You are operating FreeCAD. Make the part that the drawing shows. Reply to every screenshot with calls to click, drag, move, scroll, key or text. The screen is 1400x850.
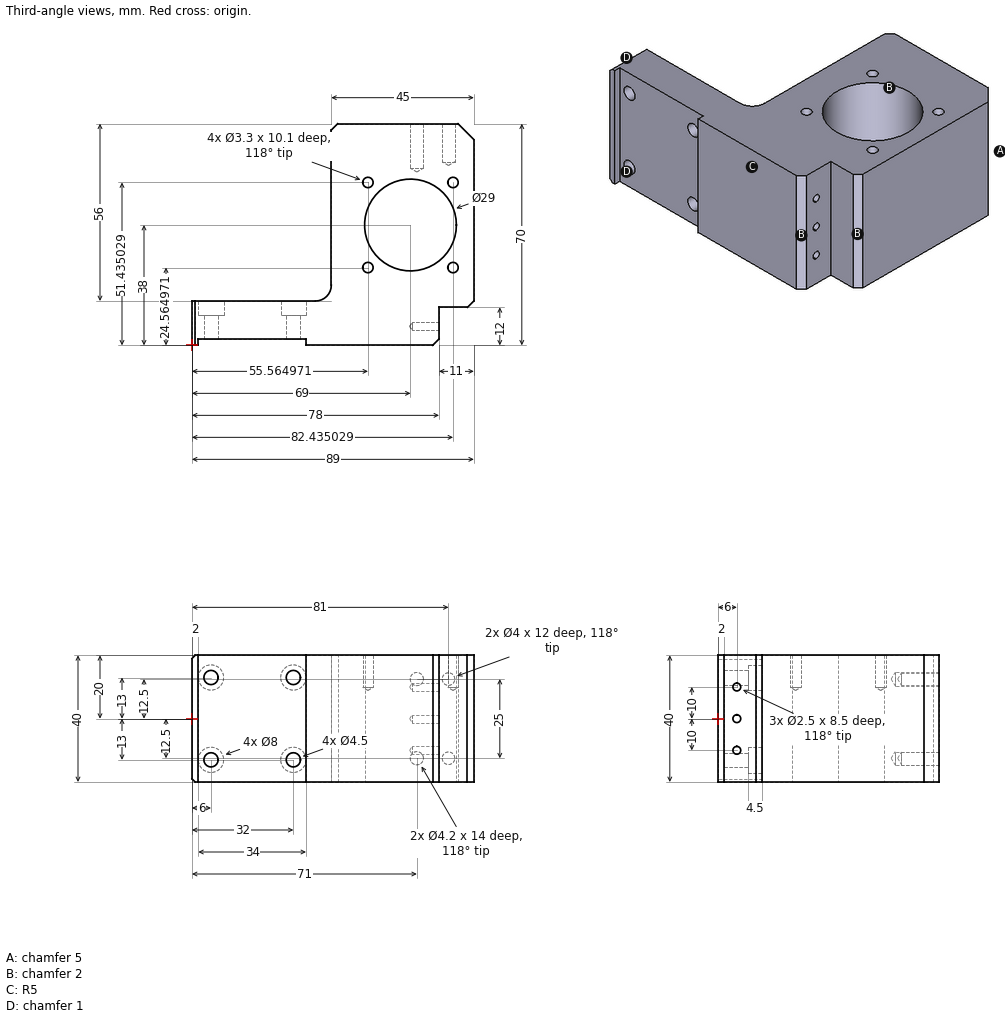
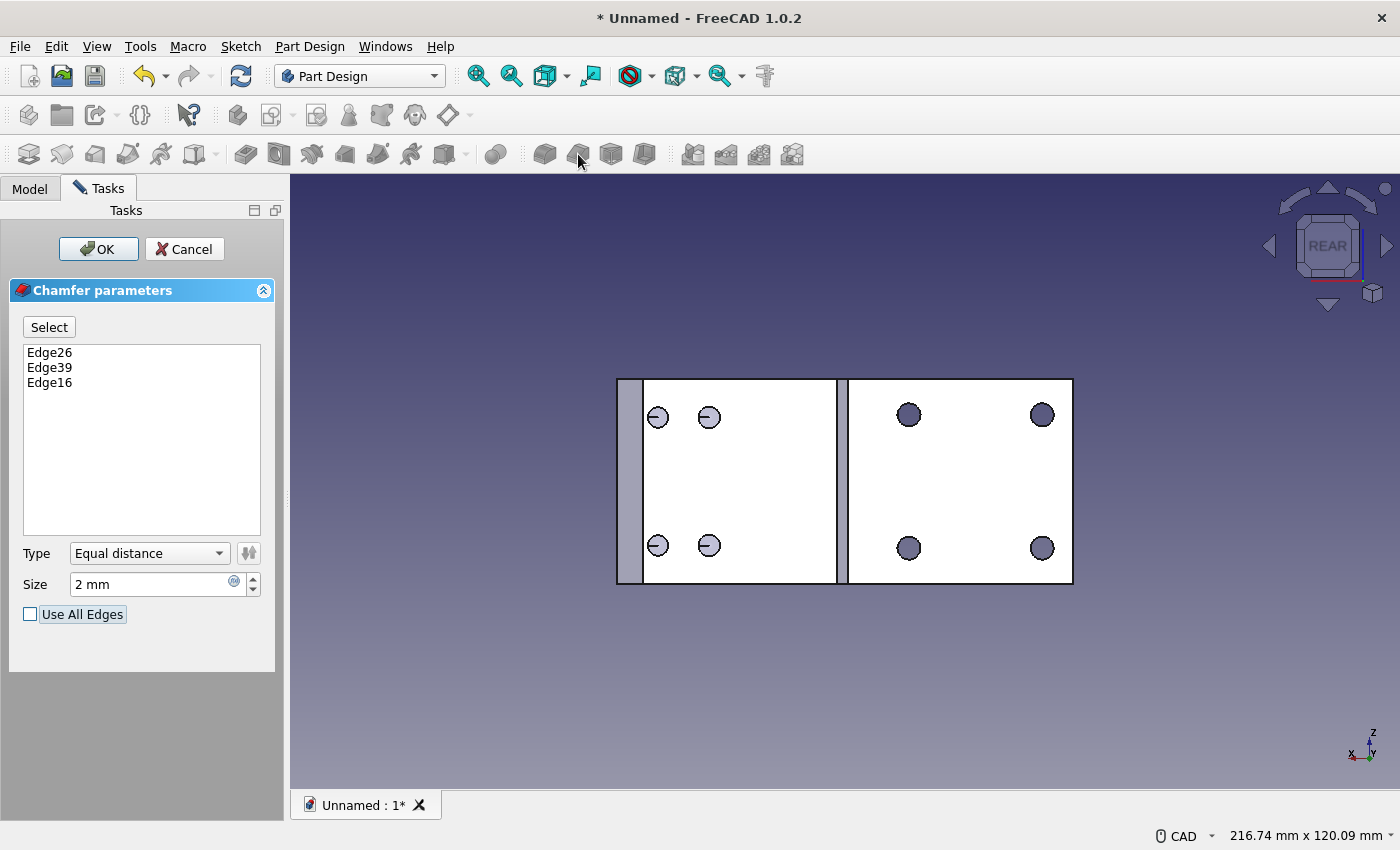
click(99, 249)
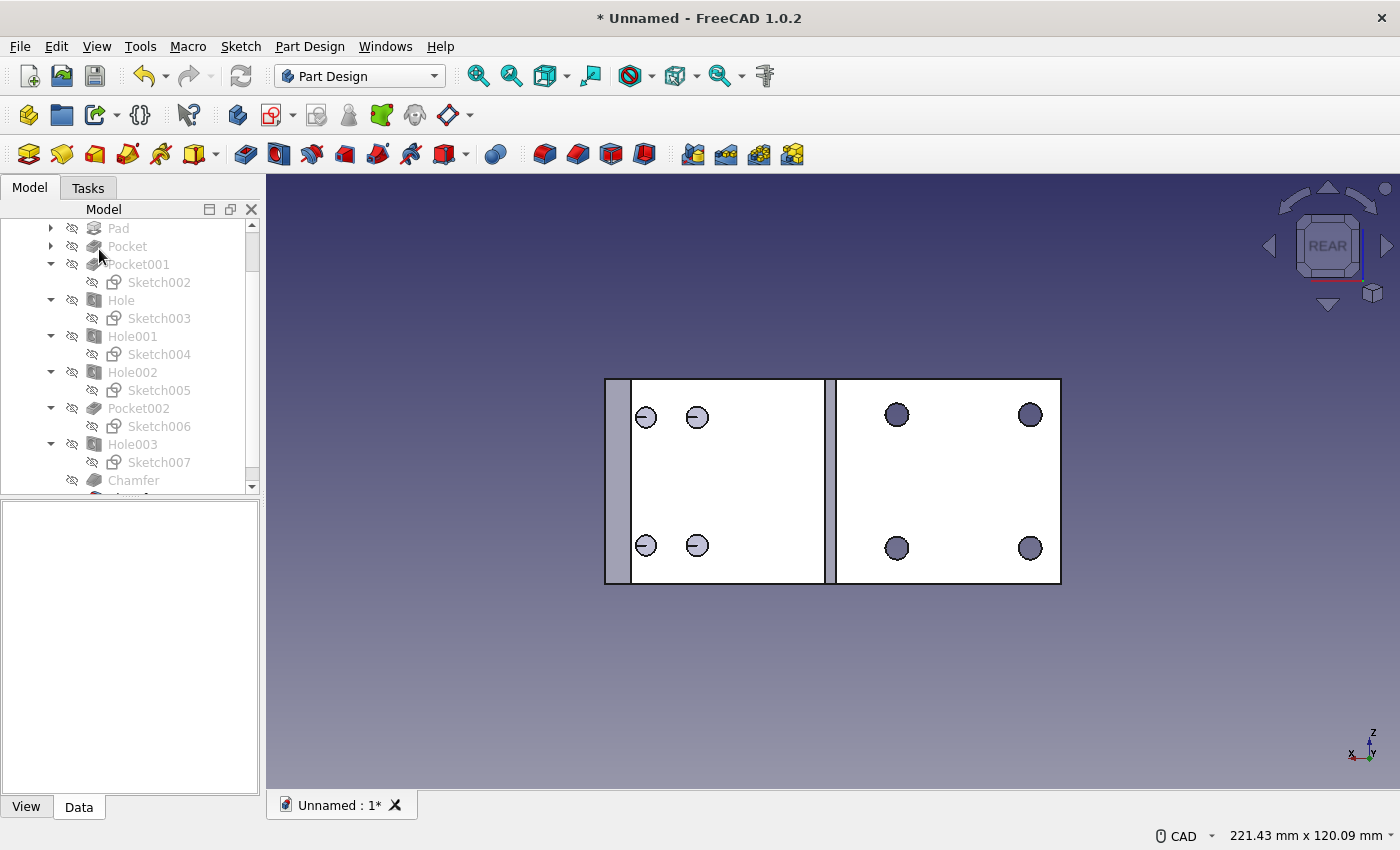
key(v)
key(f)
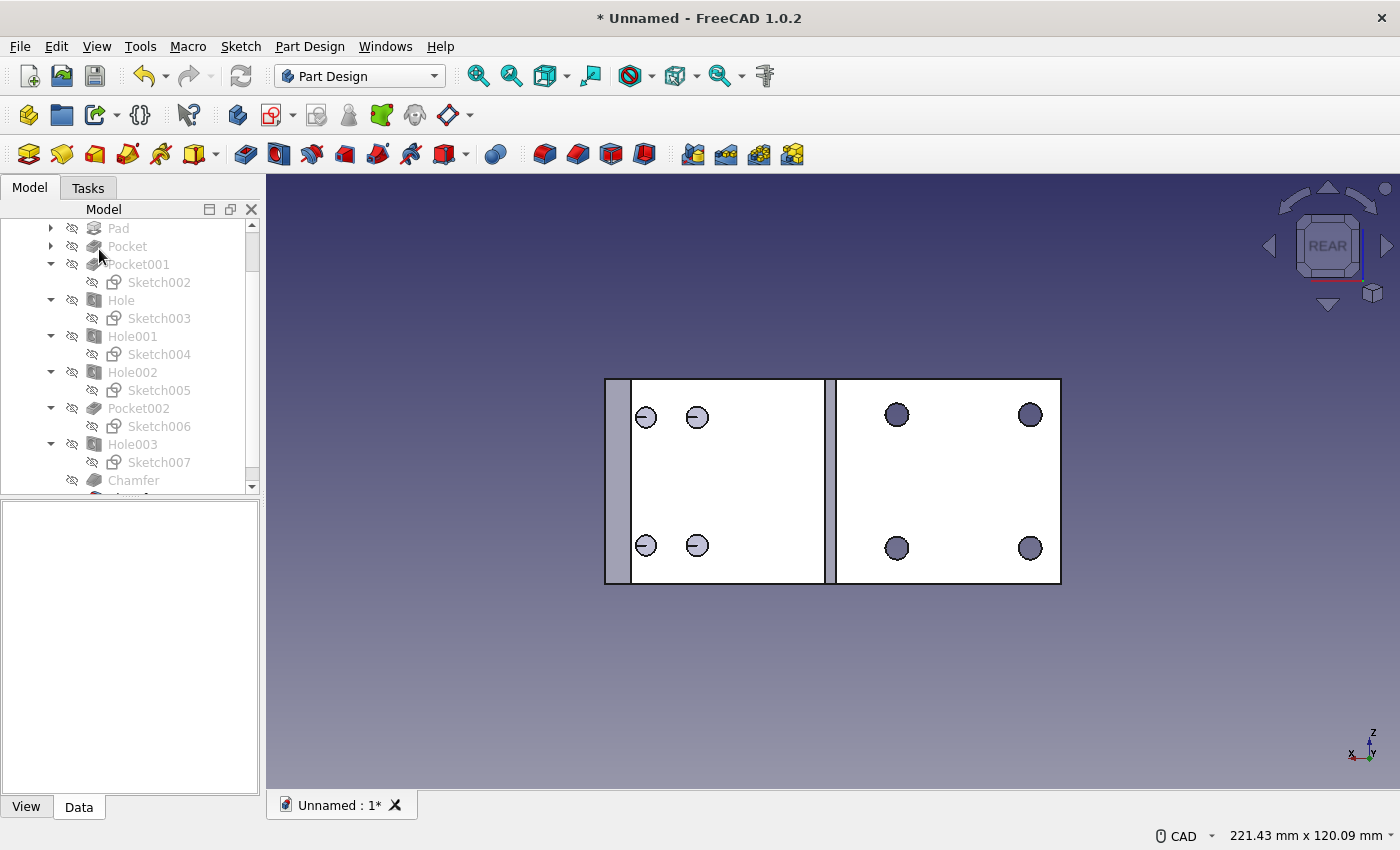
click(948, 481)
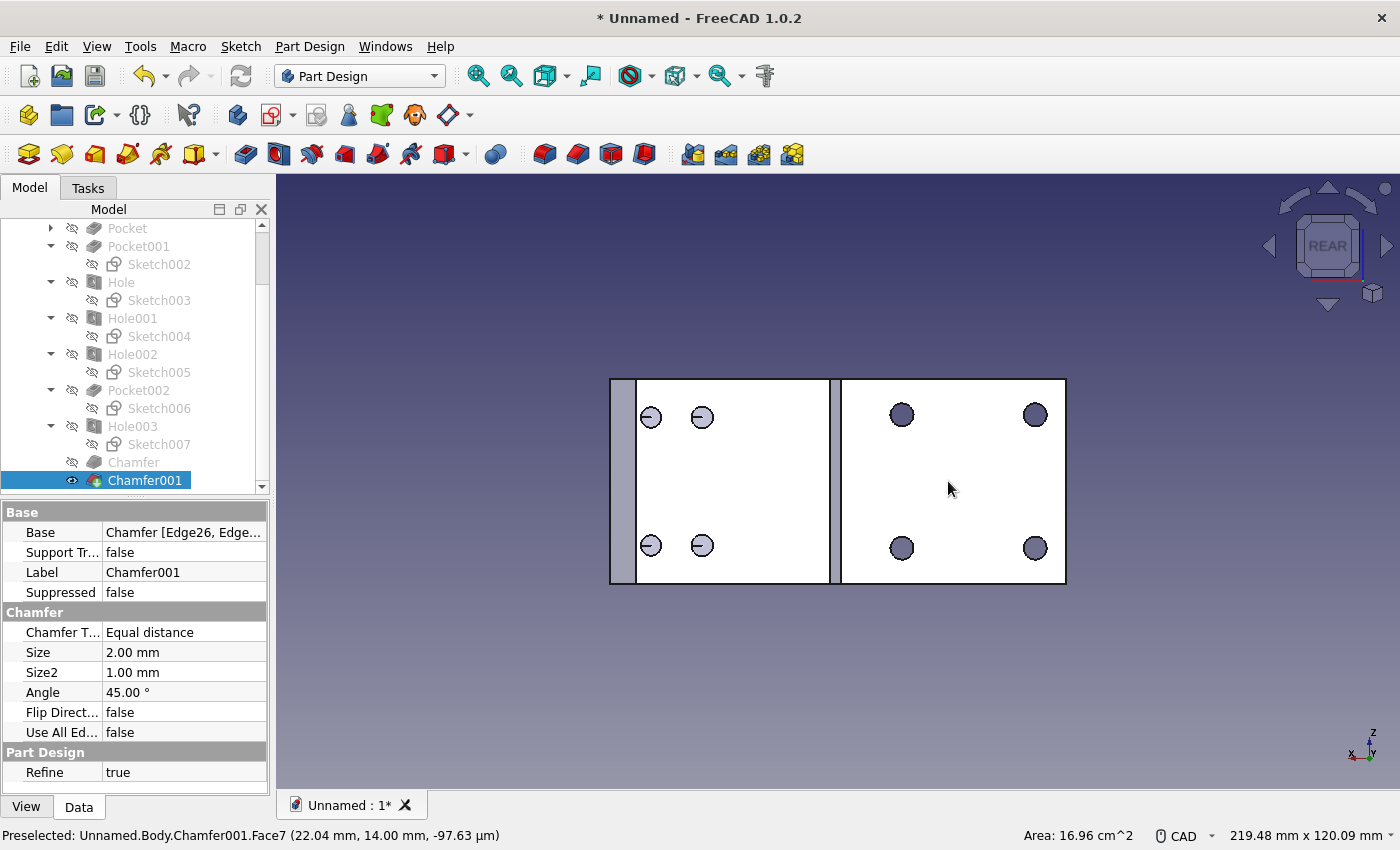
click(270, 116)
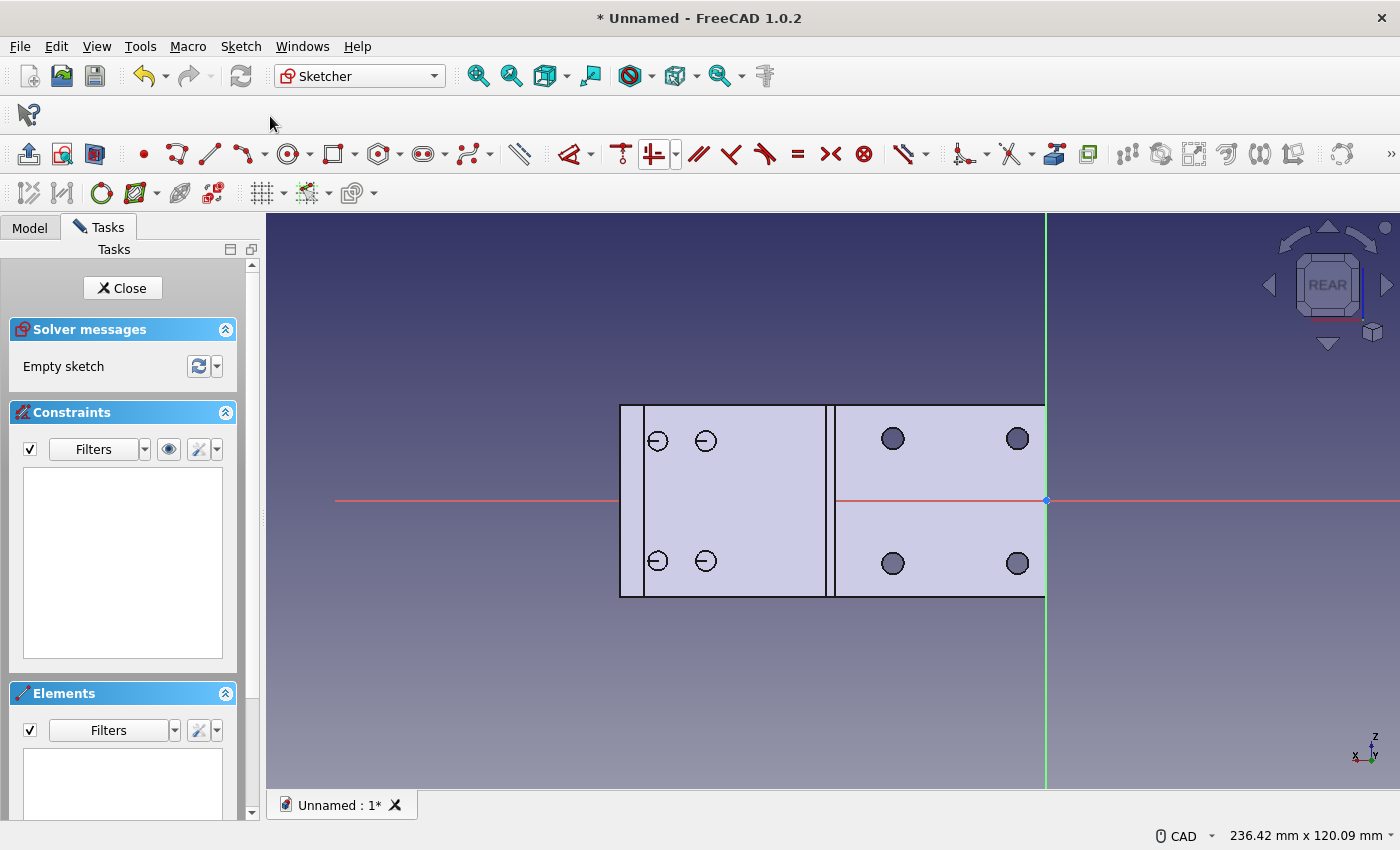
scroll(1120, 501, up, 4)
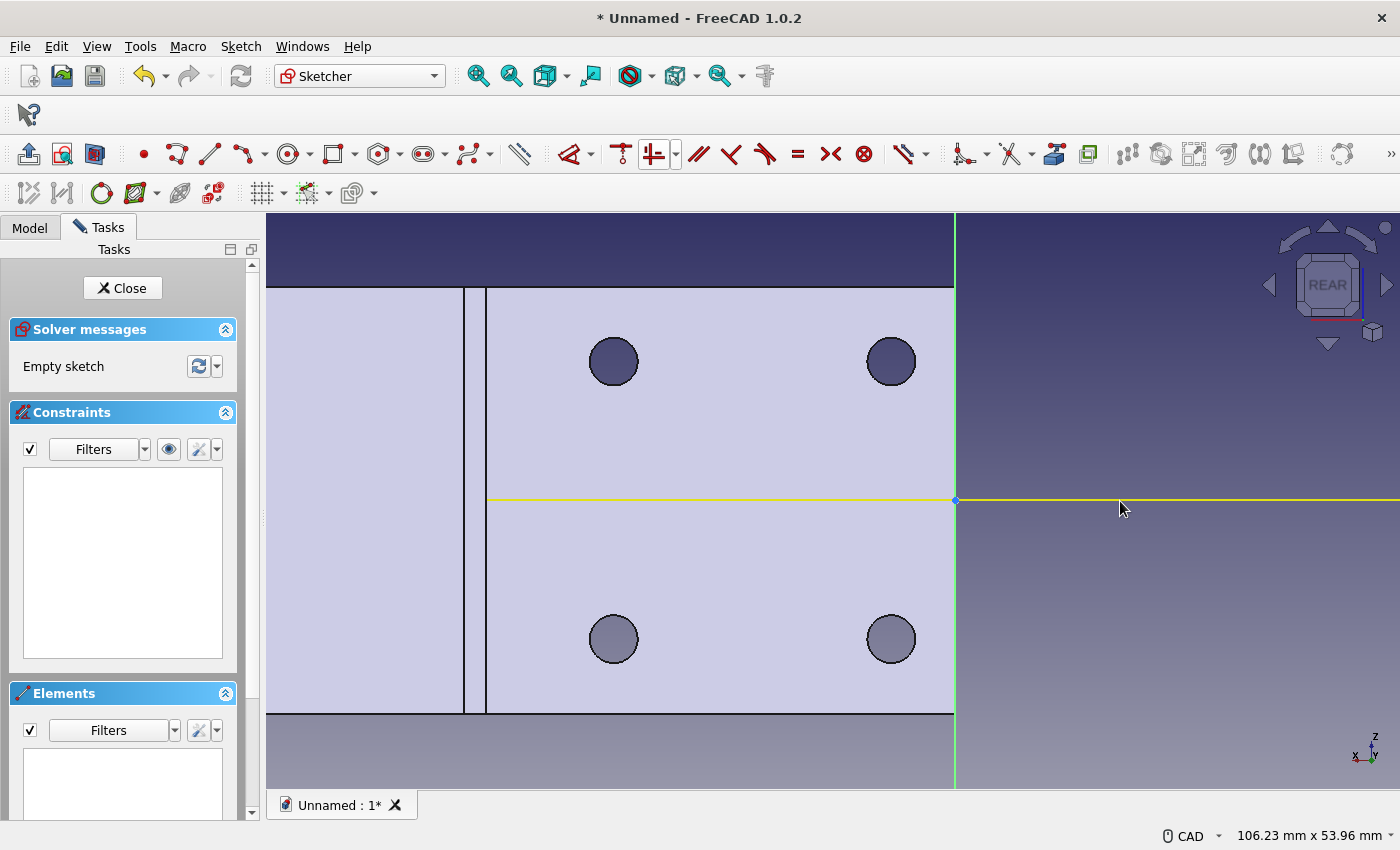
click(288, 154)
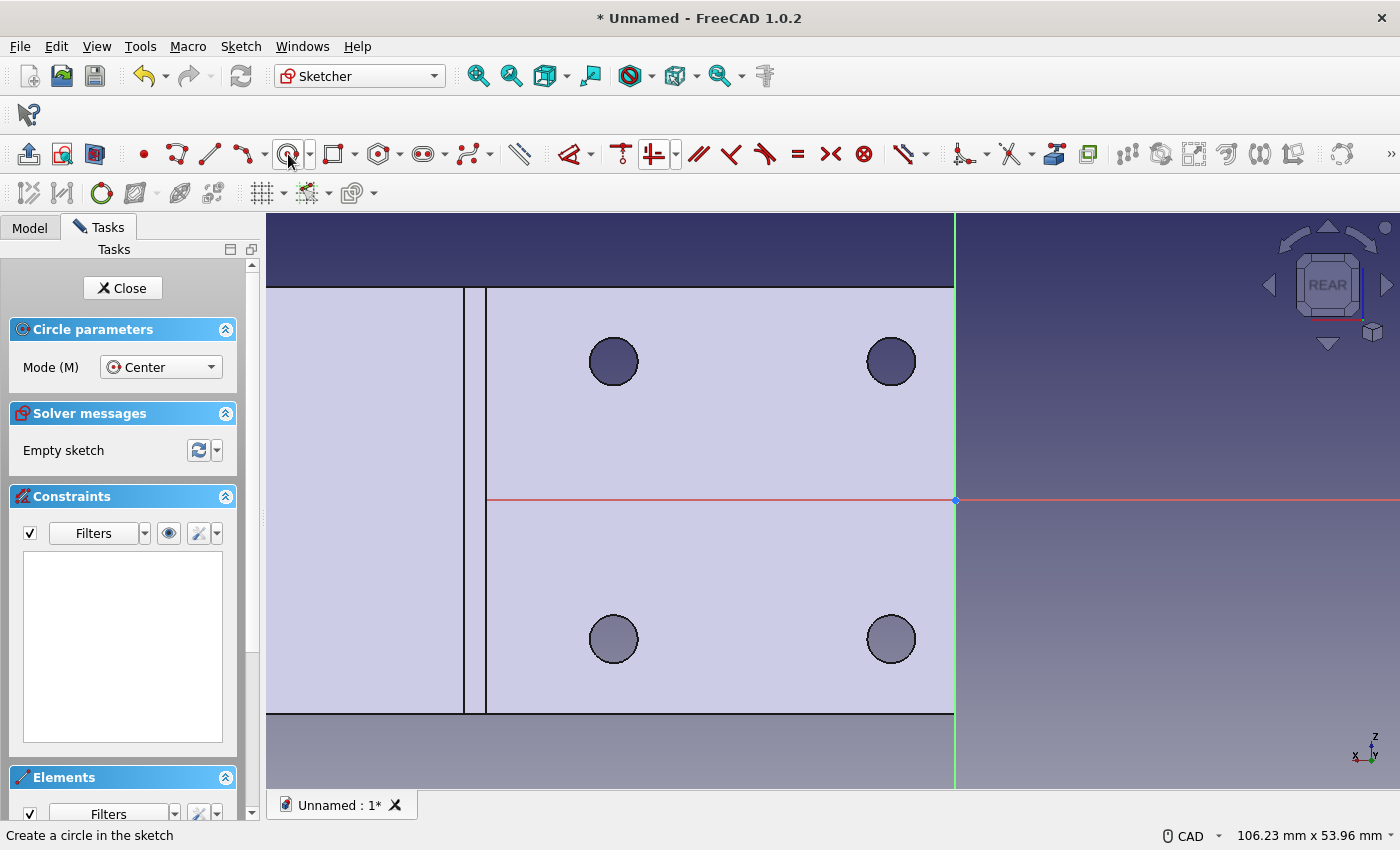
click(891, 639)
move(922, 609)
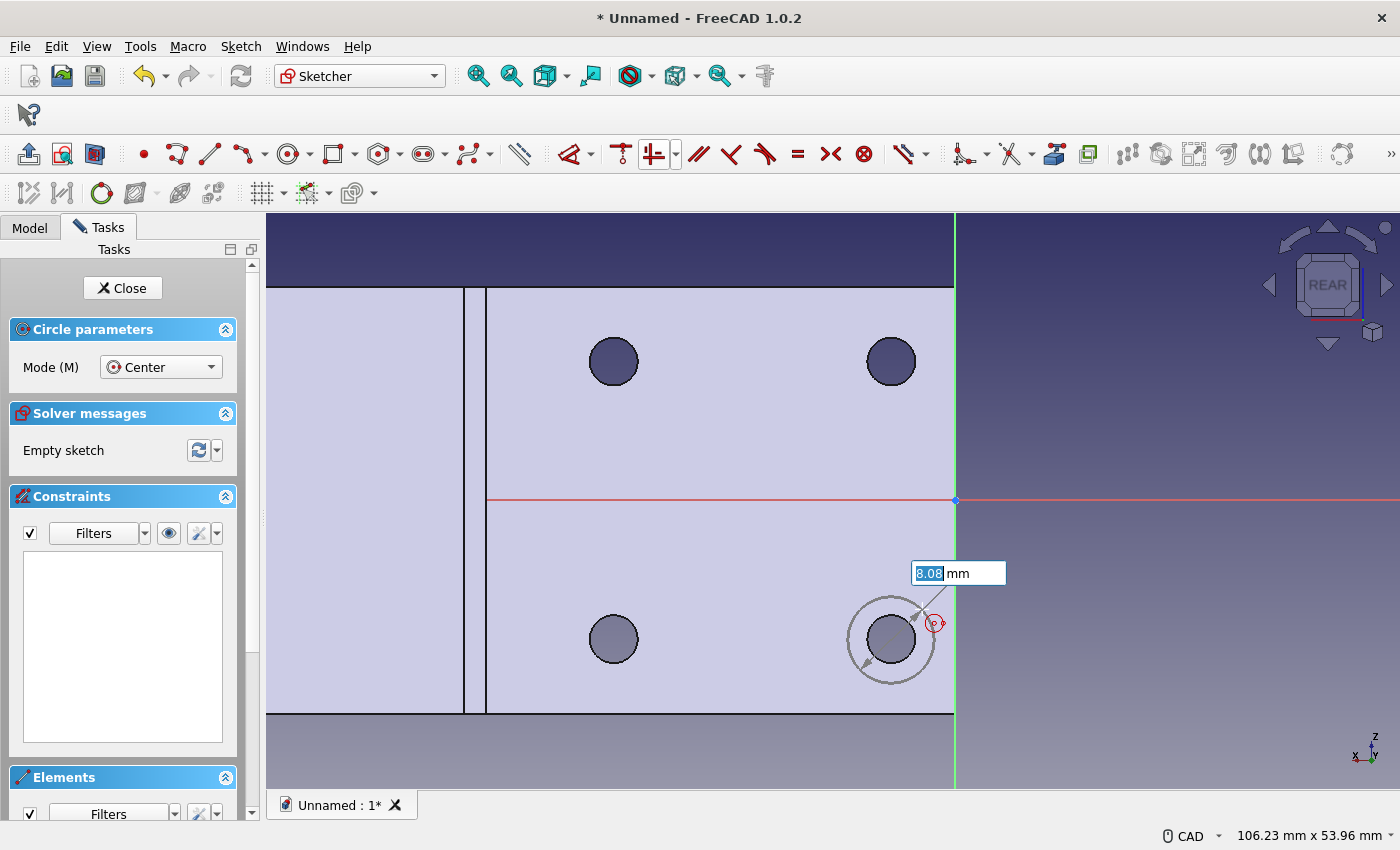
text(8)
key(Return)